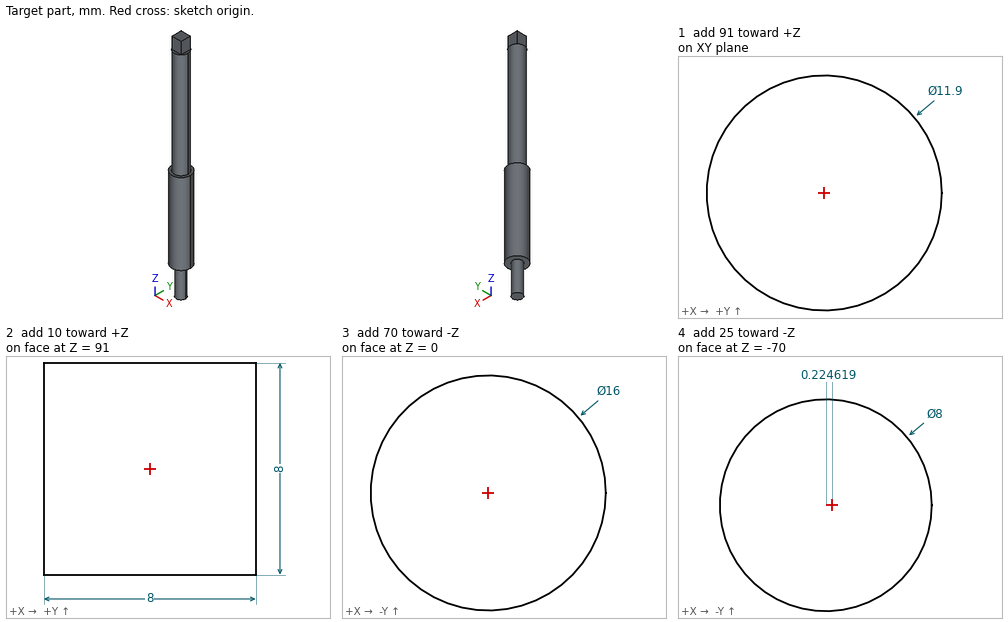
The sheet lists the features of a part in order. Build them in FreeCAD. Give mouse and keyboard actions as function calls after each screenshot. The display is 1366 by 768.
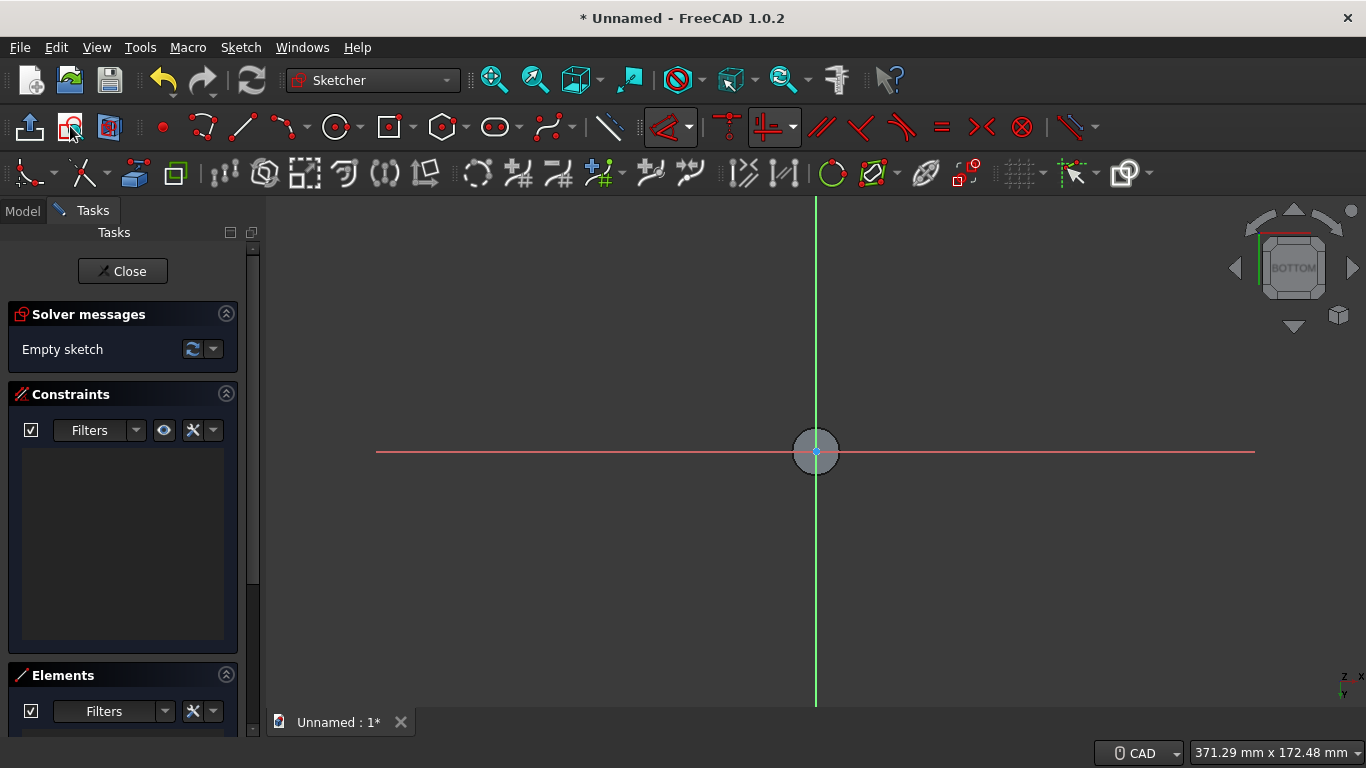
scroll(821, 452, up, 13)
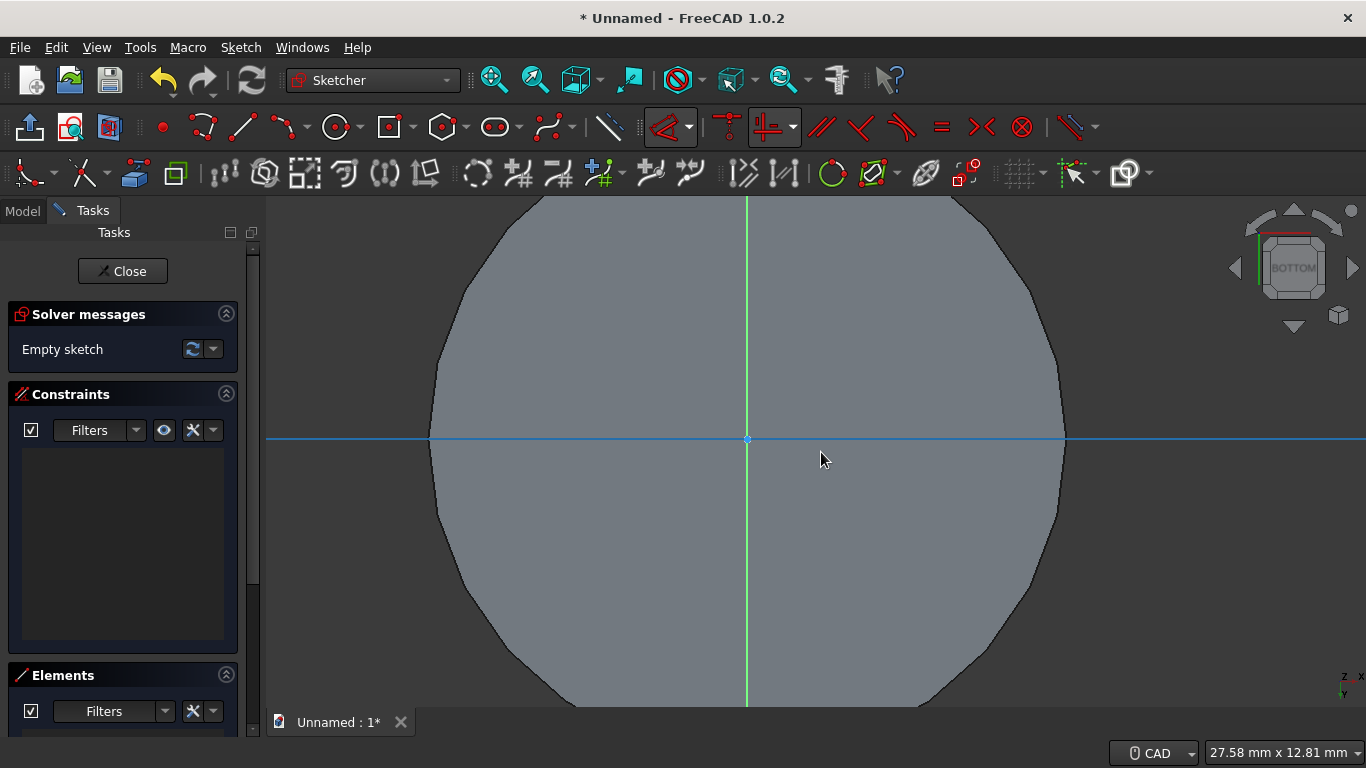
click(336, 128)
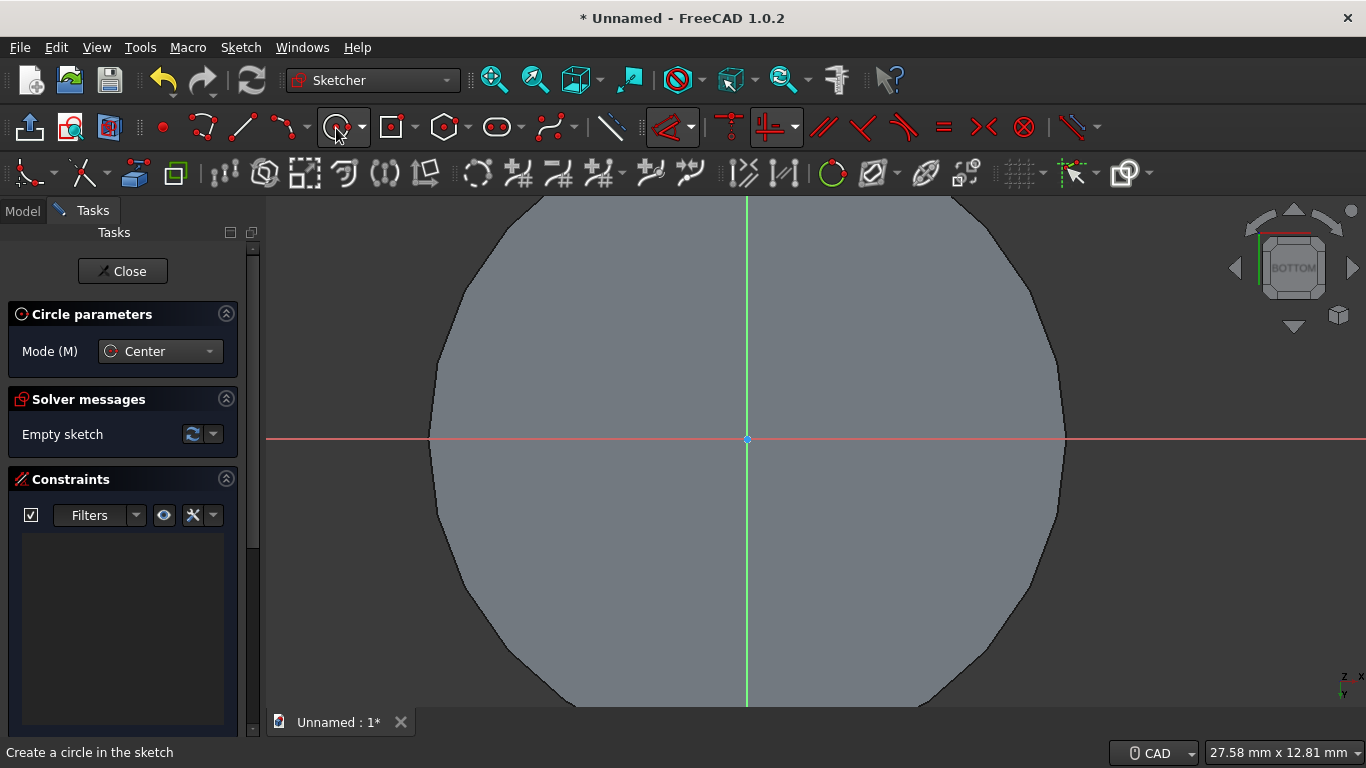
scroll(738, 439, up, 3)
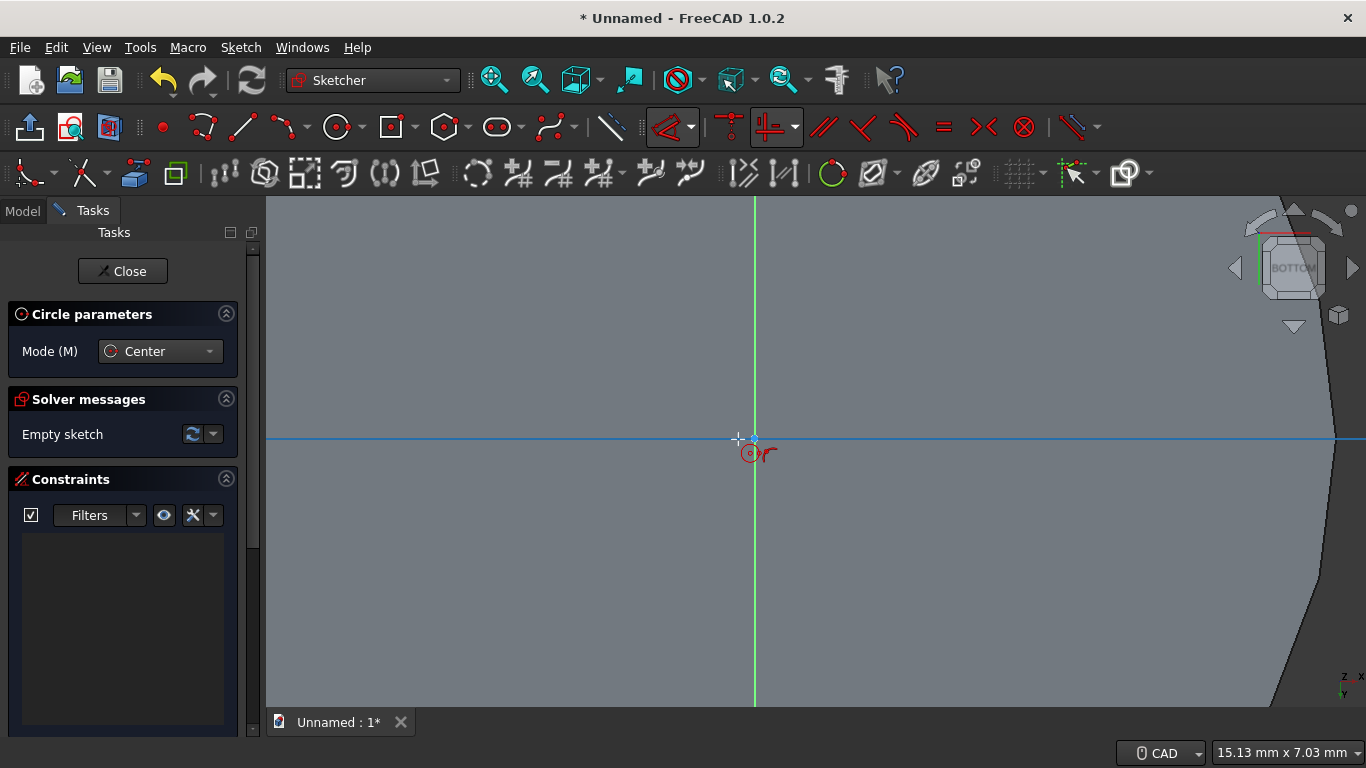
click(738, 439)
click(944, 233)
key(Escape)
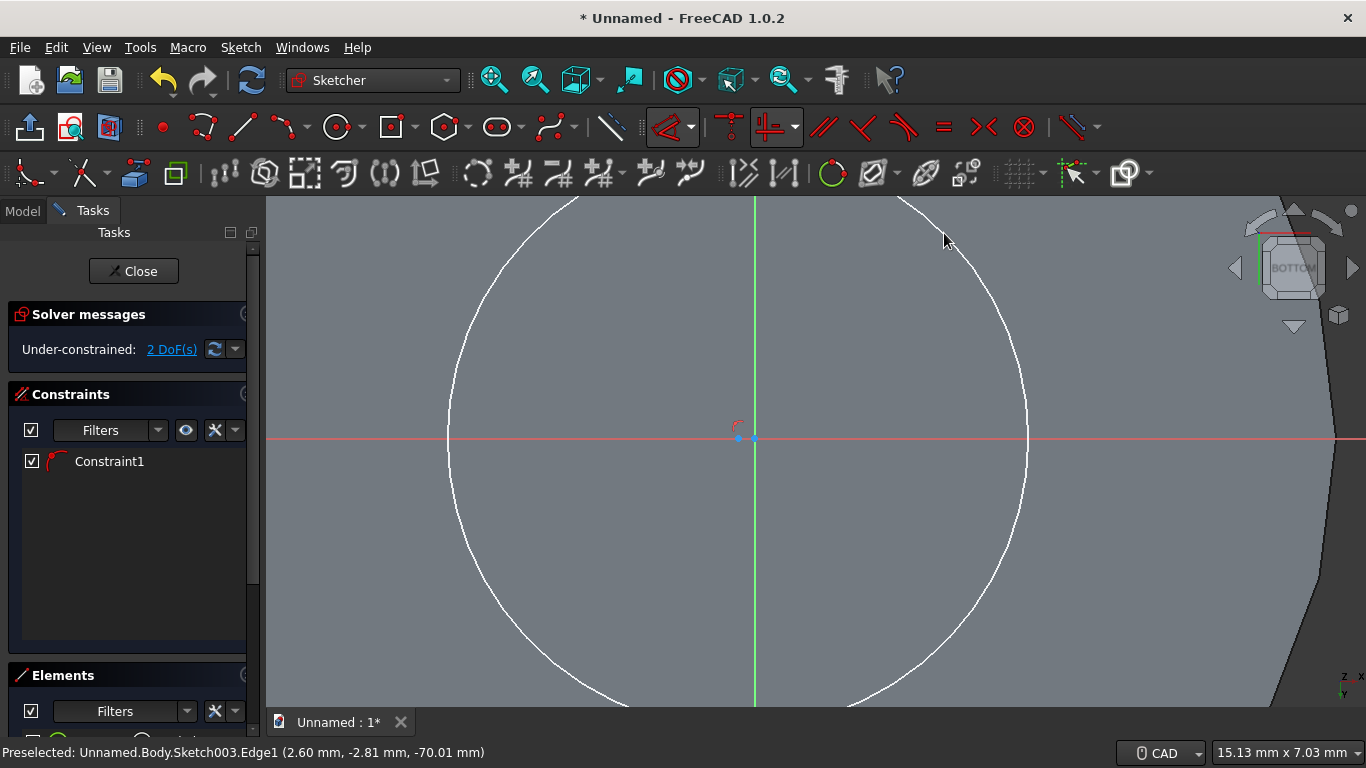
click(943, 233)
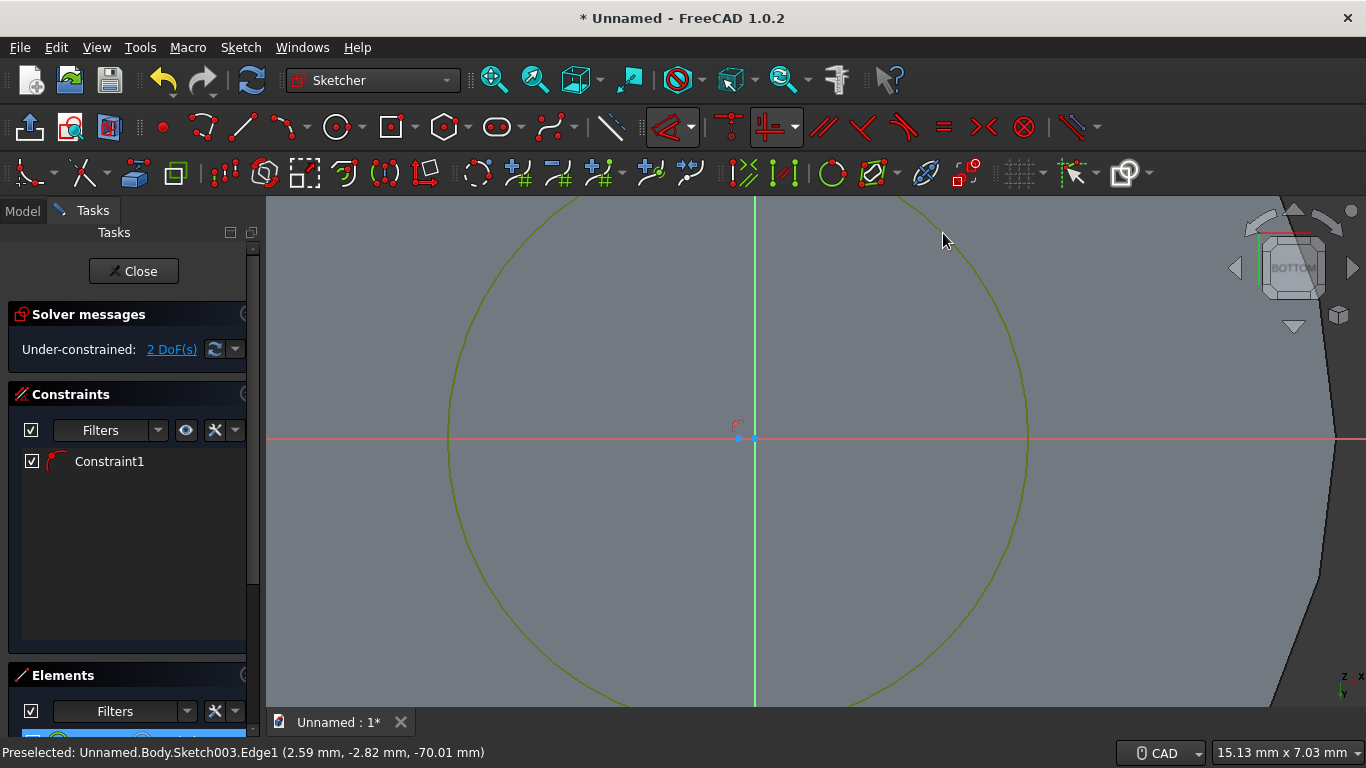
key(k)
key(o)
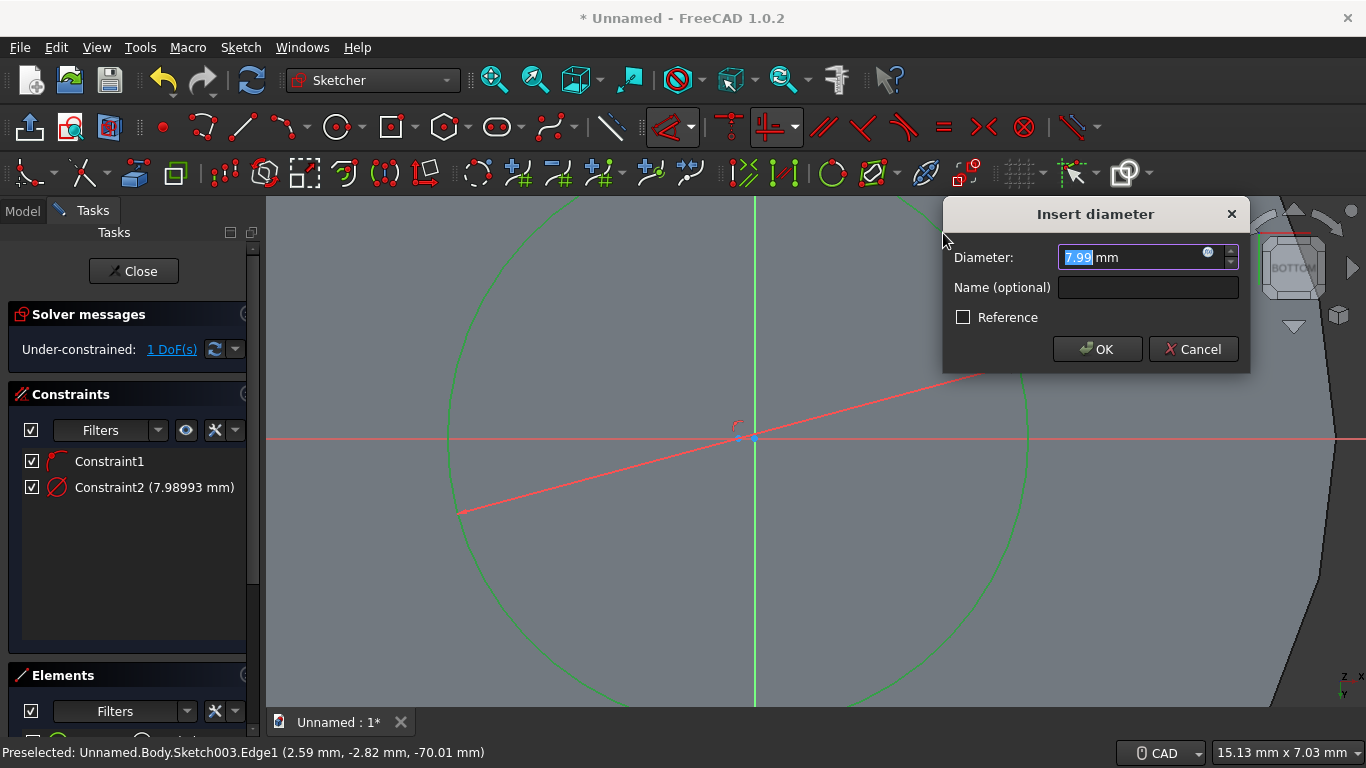
text(8)
key(Return)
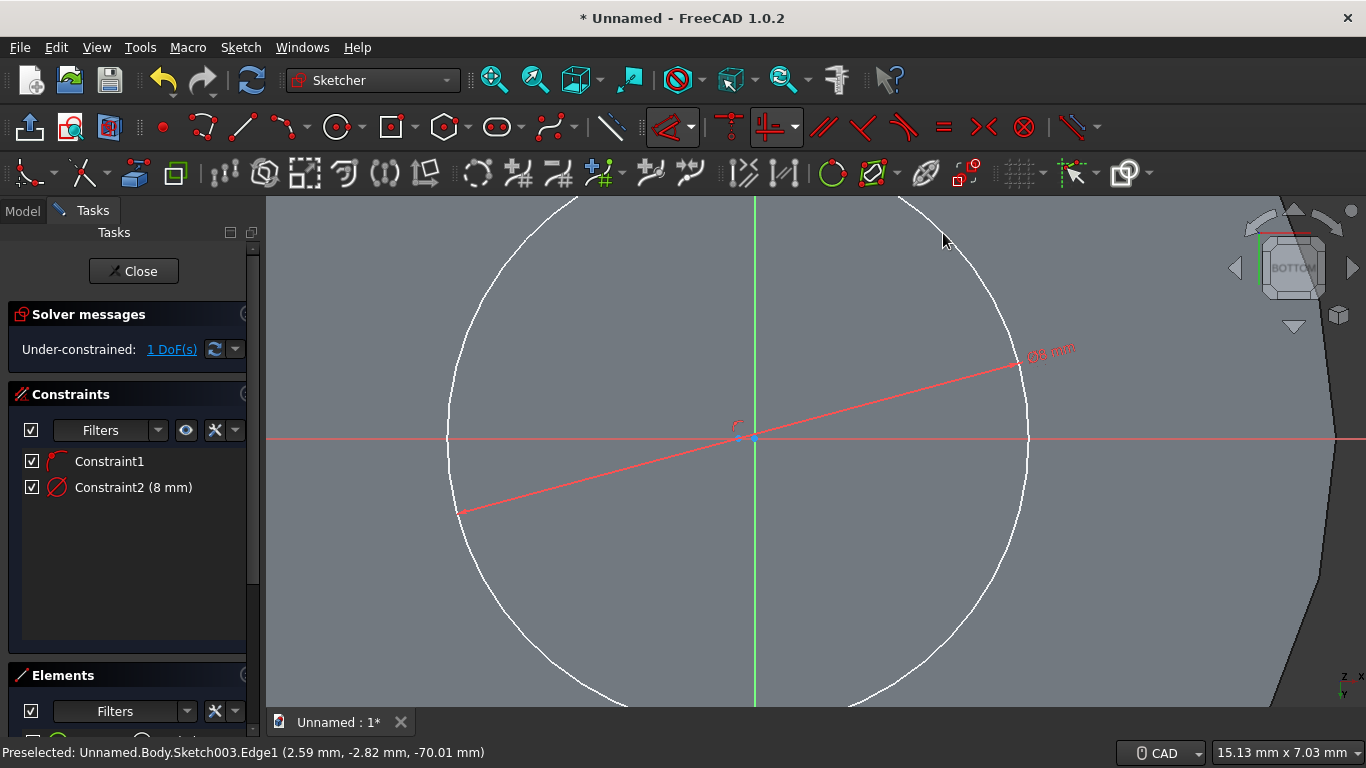
scroll(738, 439, up, 5)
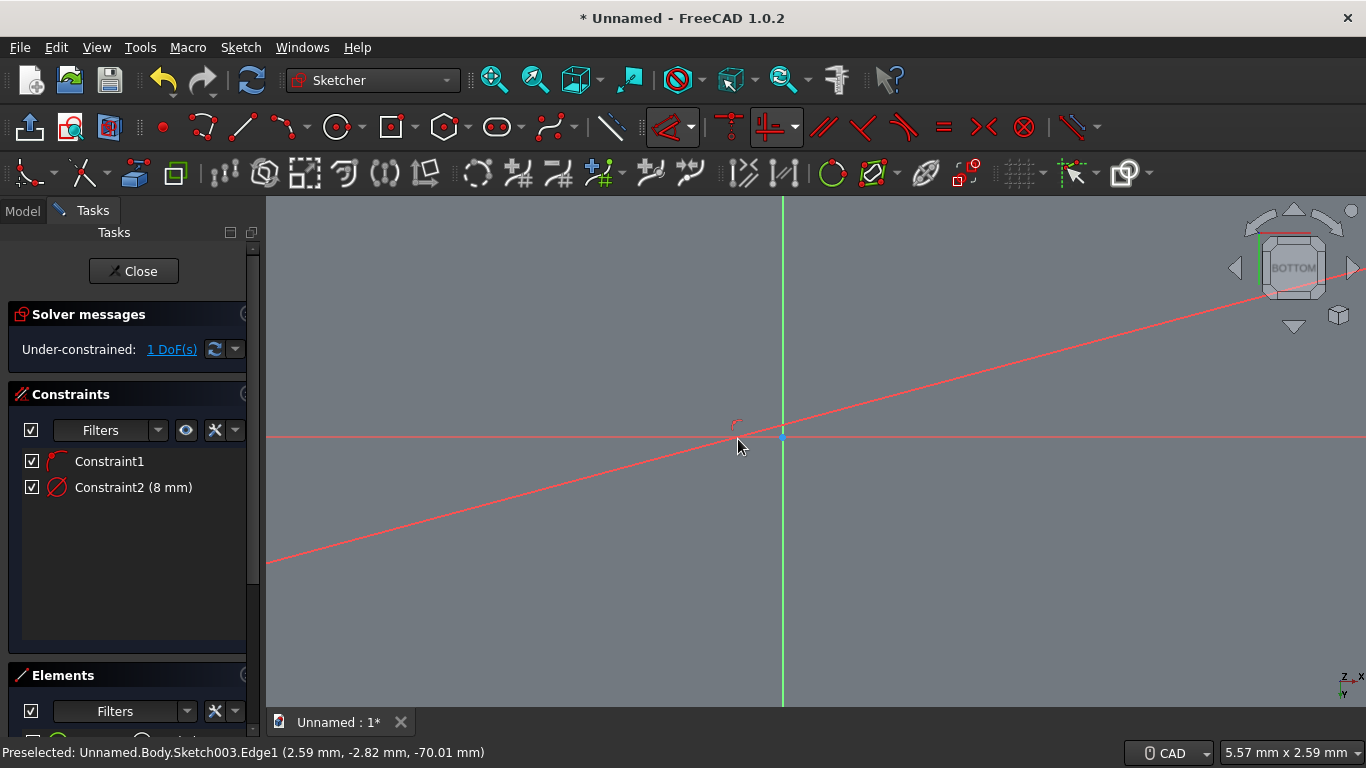
click(737, 437)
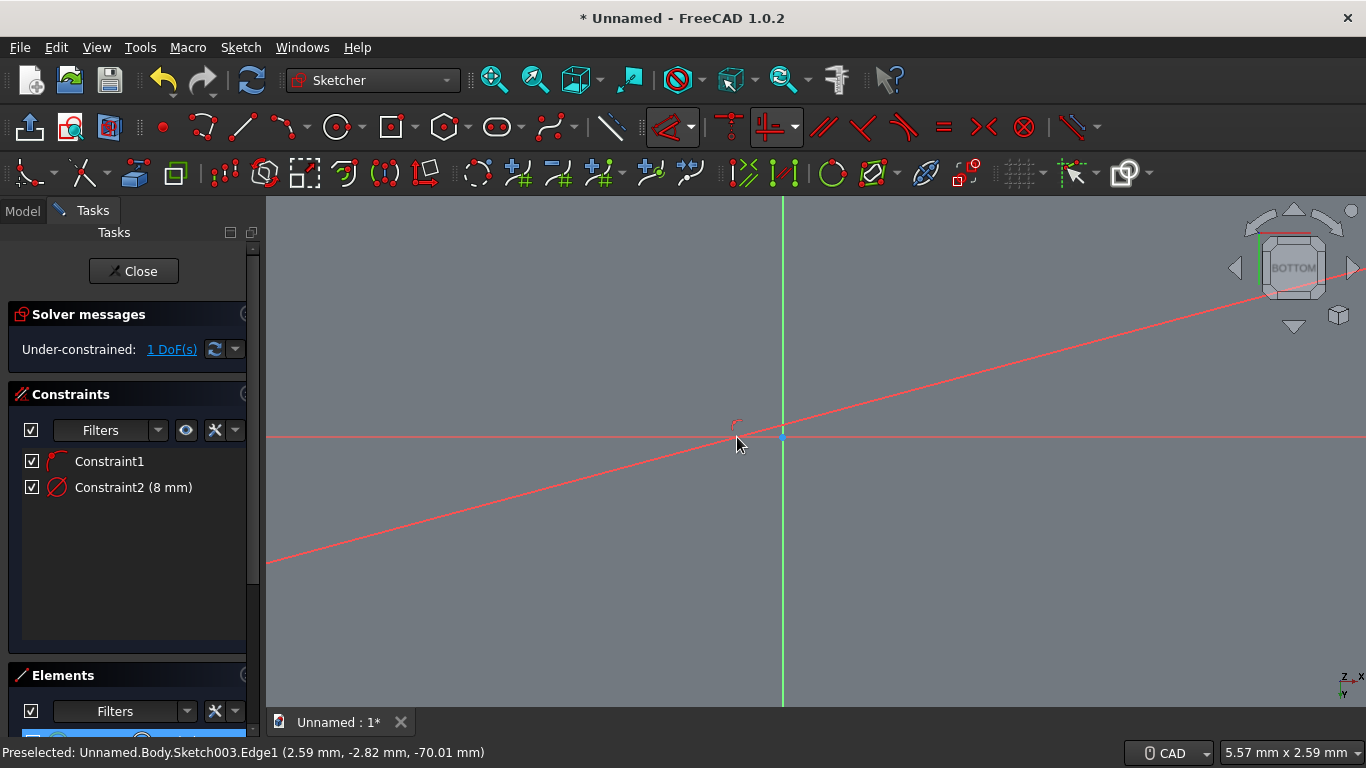
key(l)